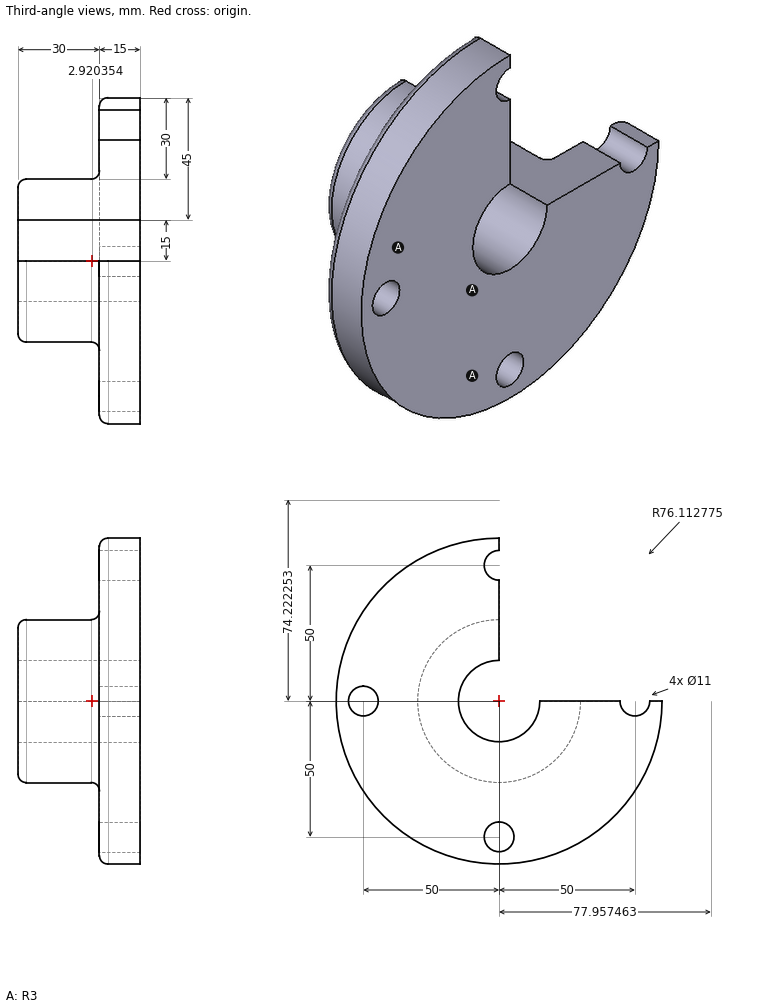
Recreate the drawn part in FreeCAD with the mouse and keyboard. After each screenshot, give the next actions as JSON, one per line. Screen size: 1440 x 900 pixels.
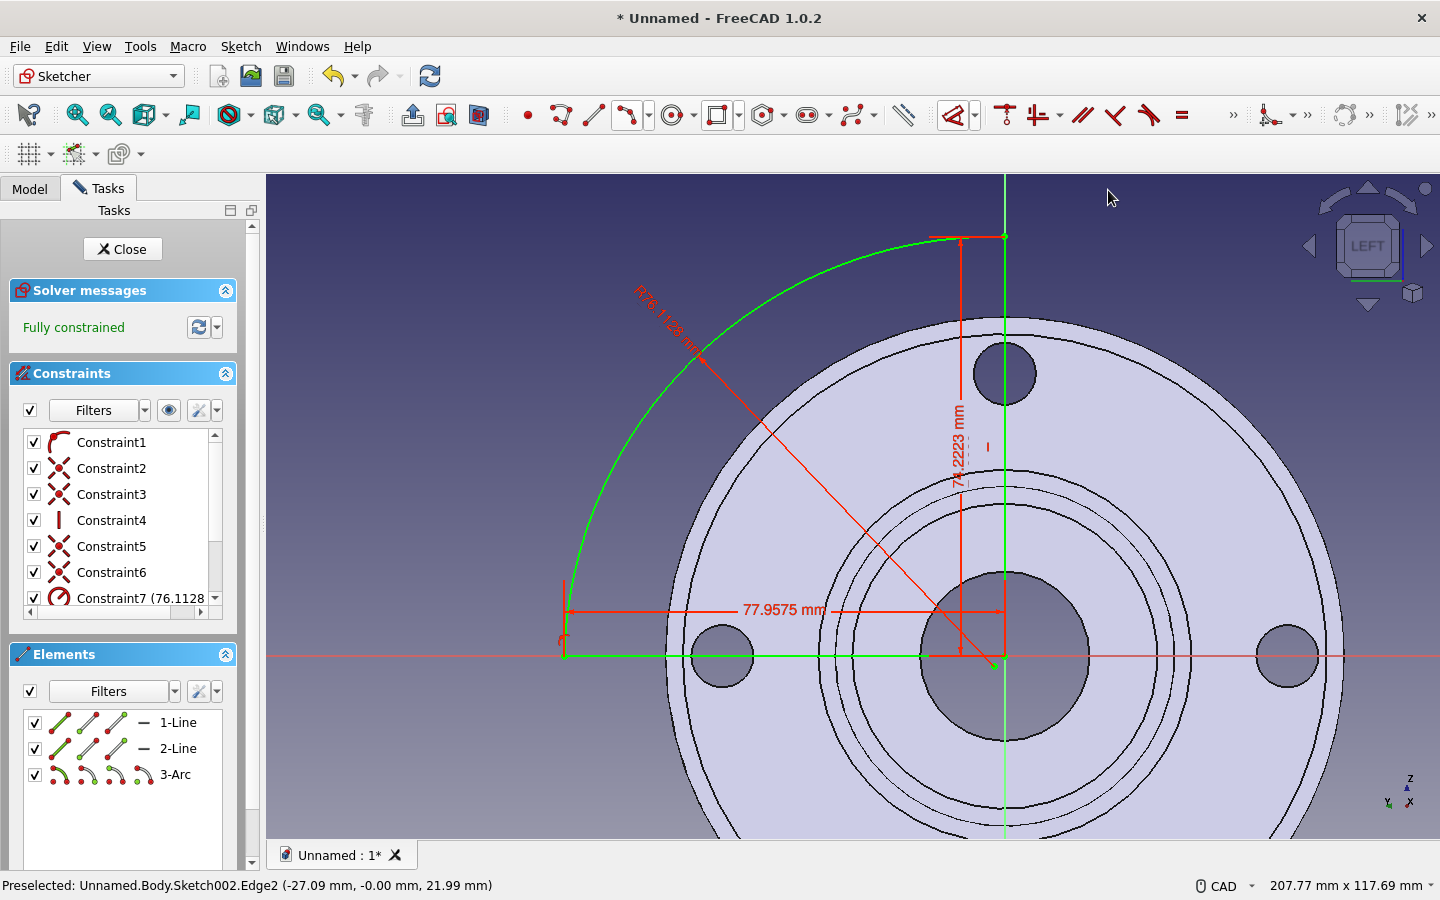
{"action": "left_click", "coordinate": [123, 249]}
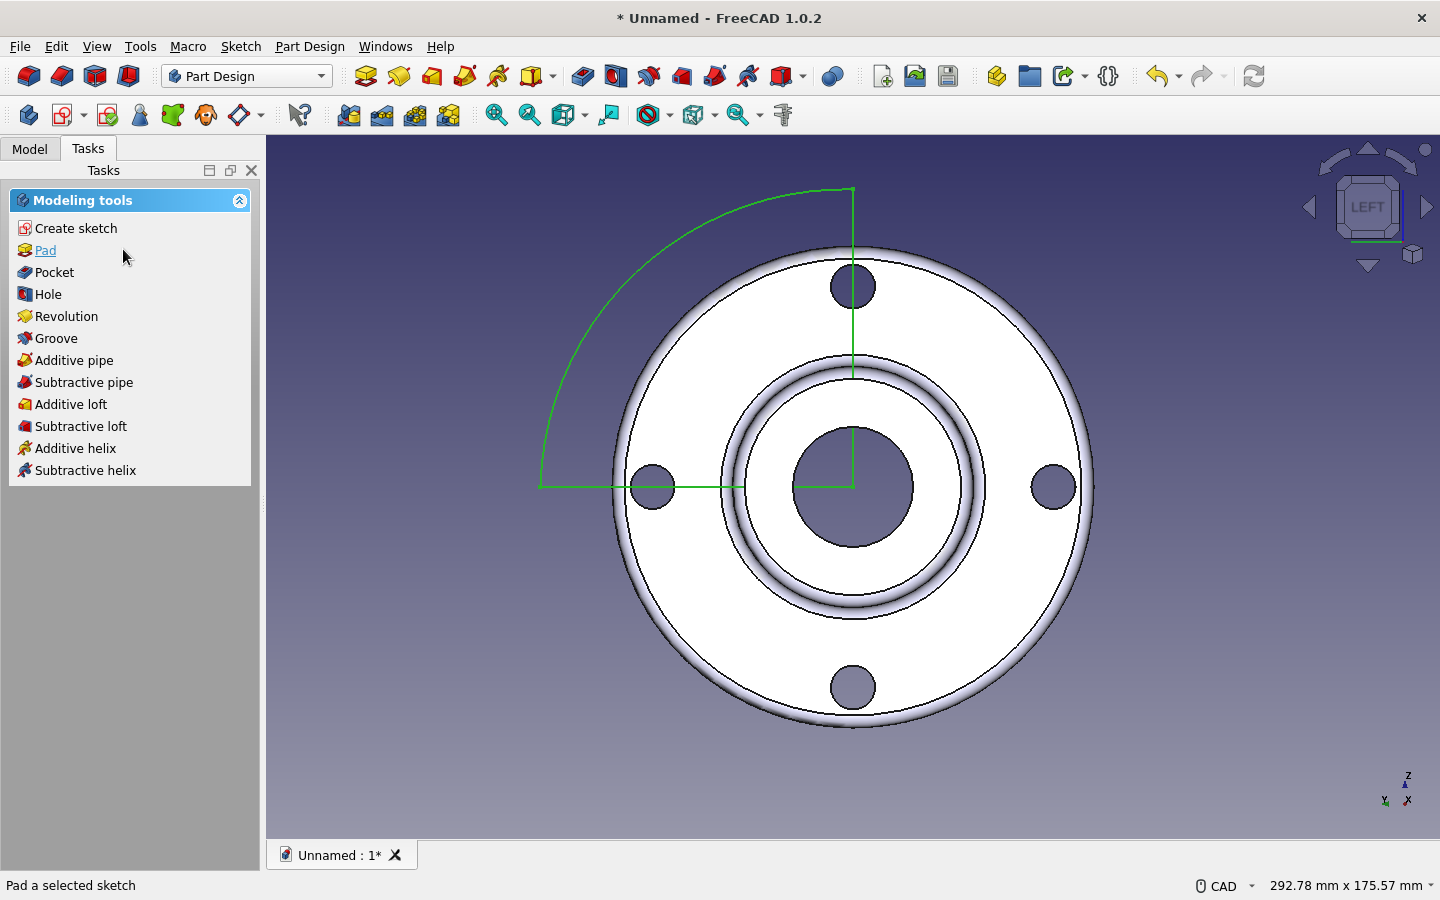
{"action": "left_click", "coordinate": [583, 76]}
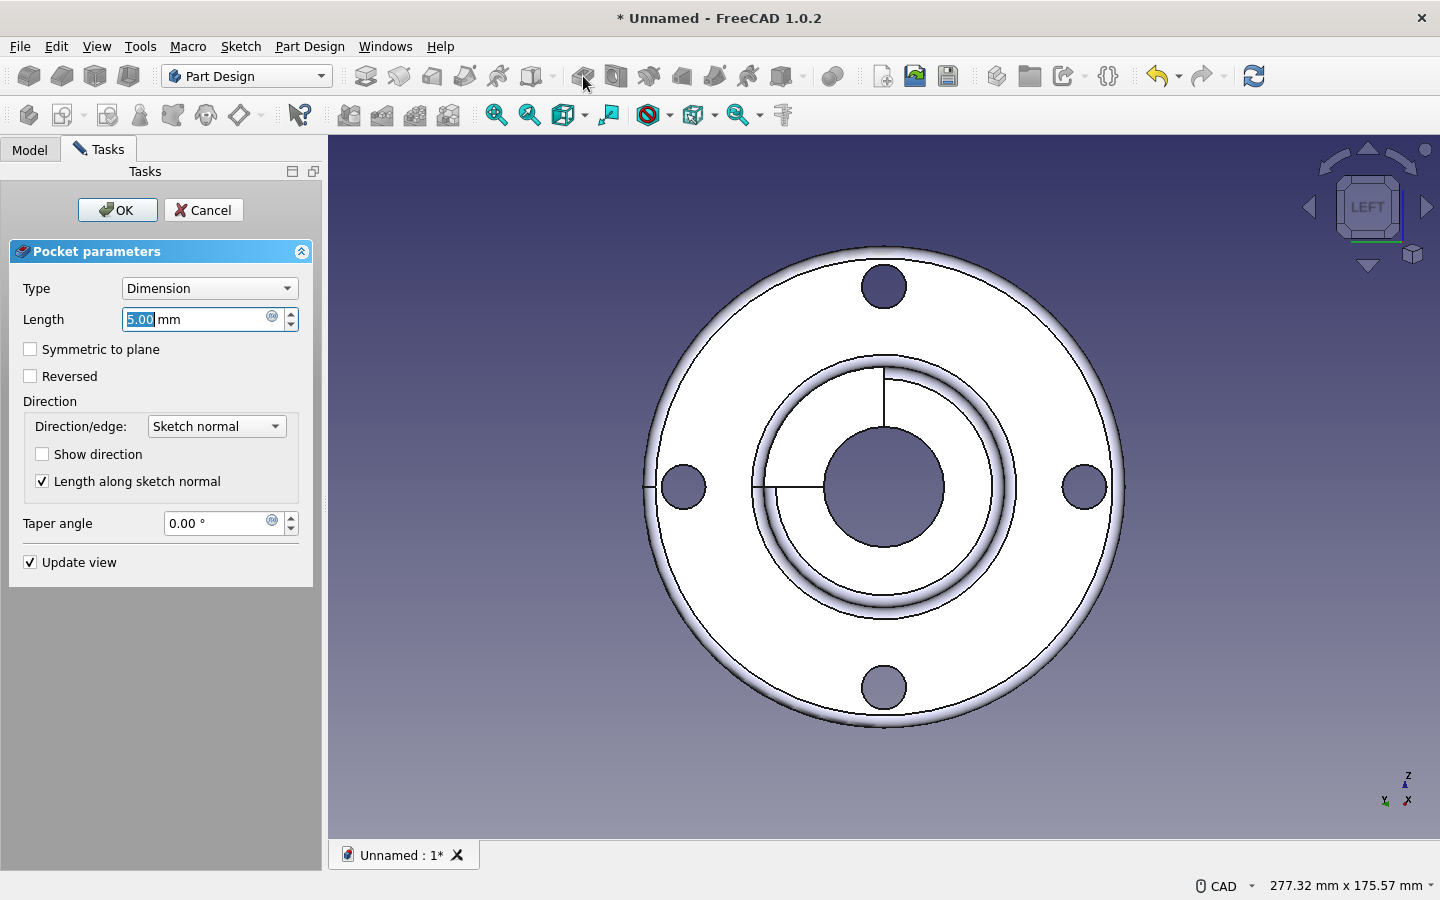
{"action": "left_click", "coordinate": [210, 288]}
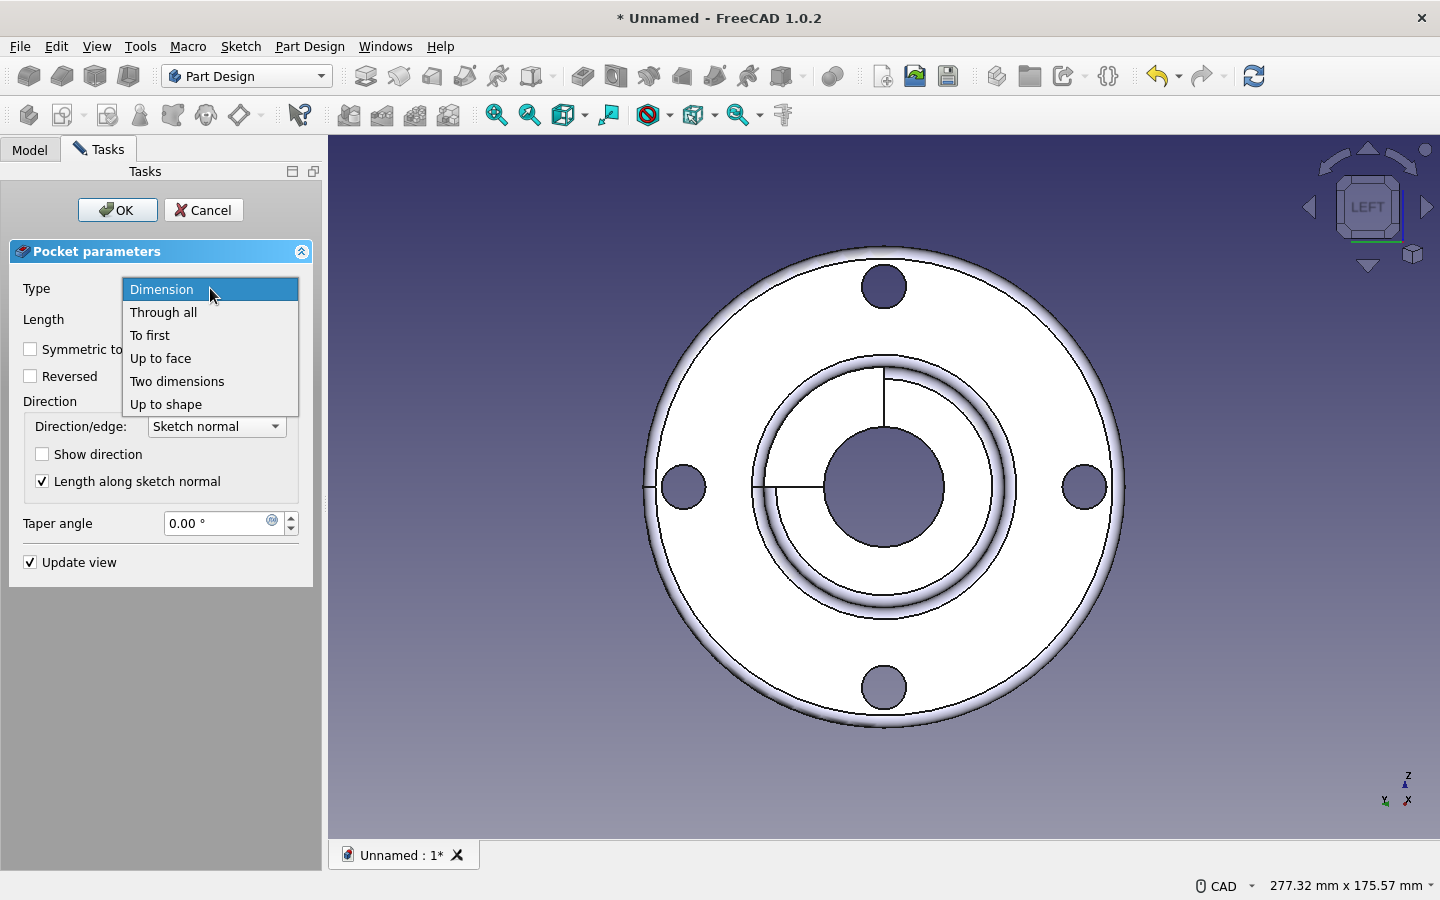
{"action": "left_click", "coordinate": [208, 312]}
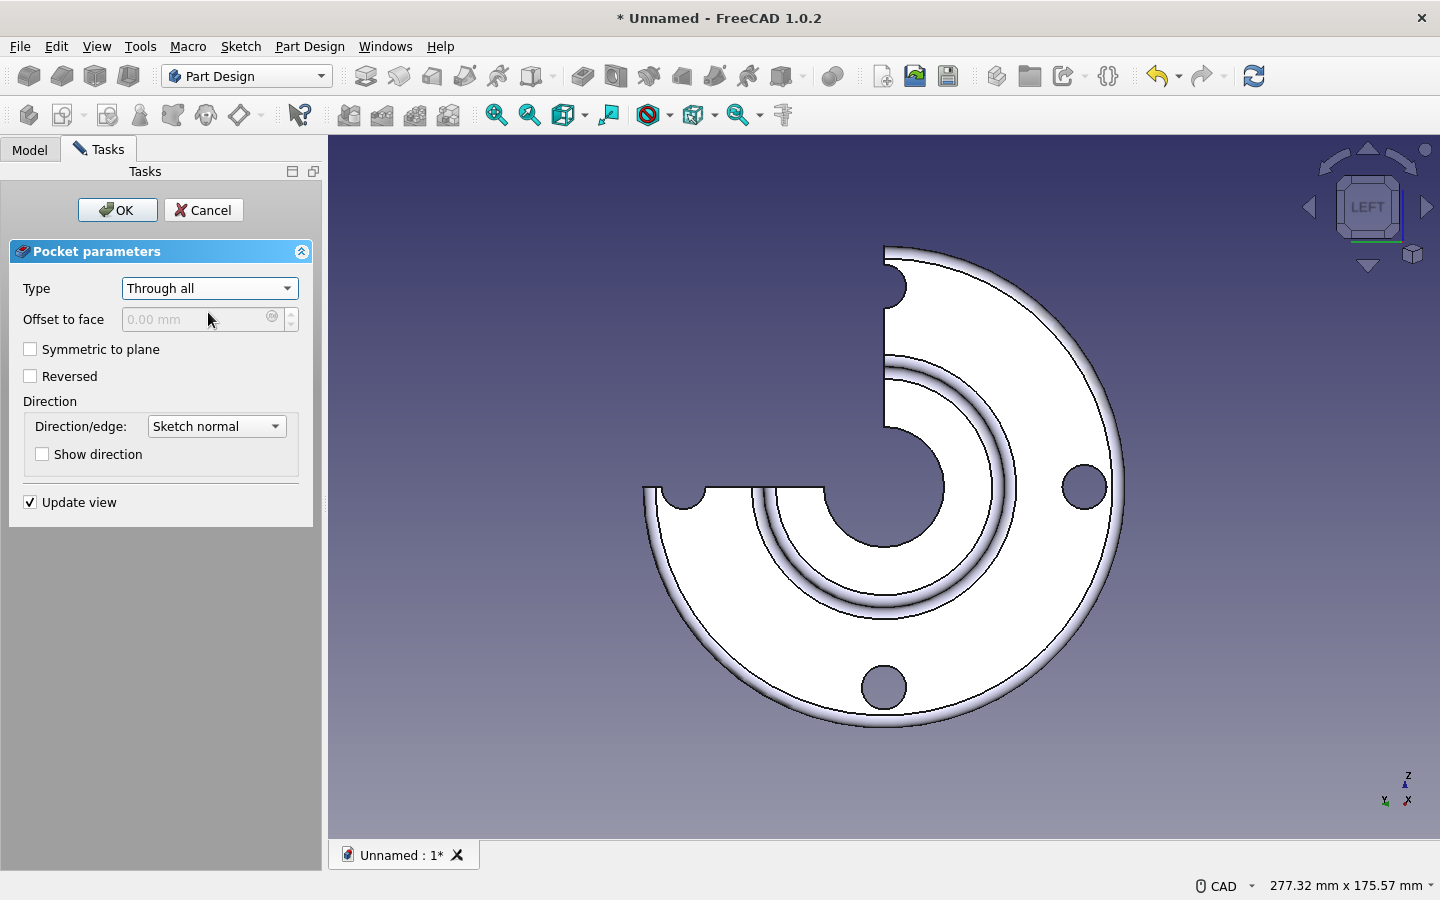
{"action": "left_click", "coordinate": [118, 210]}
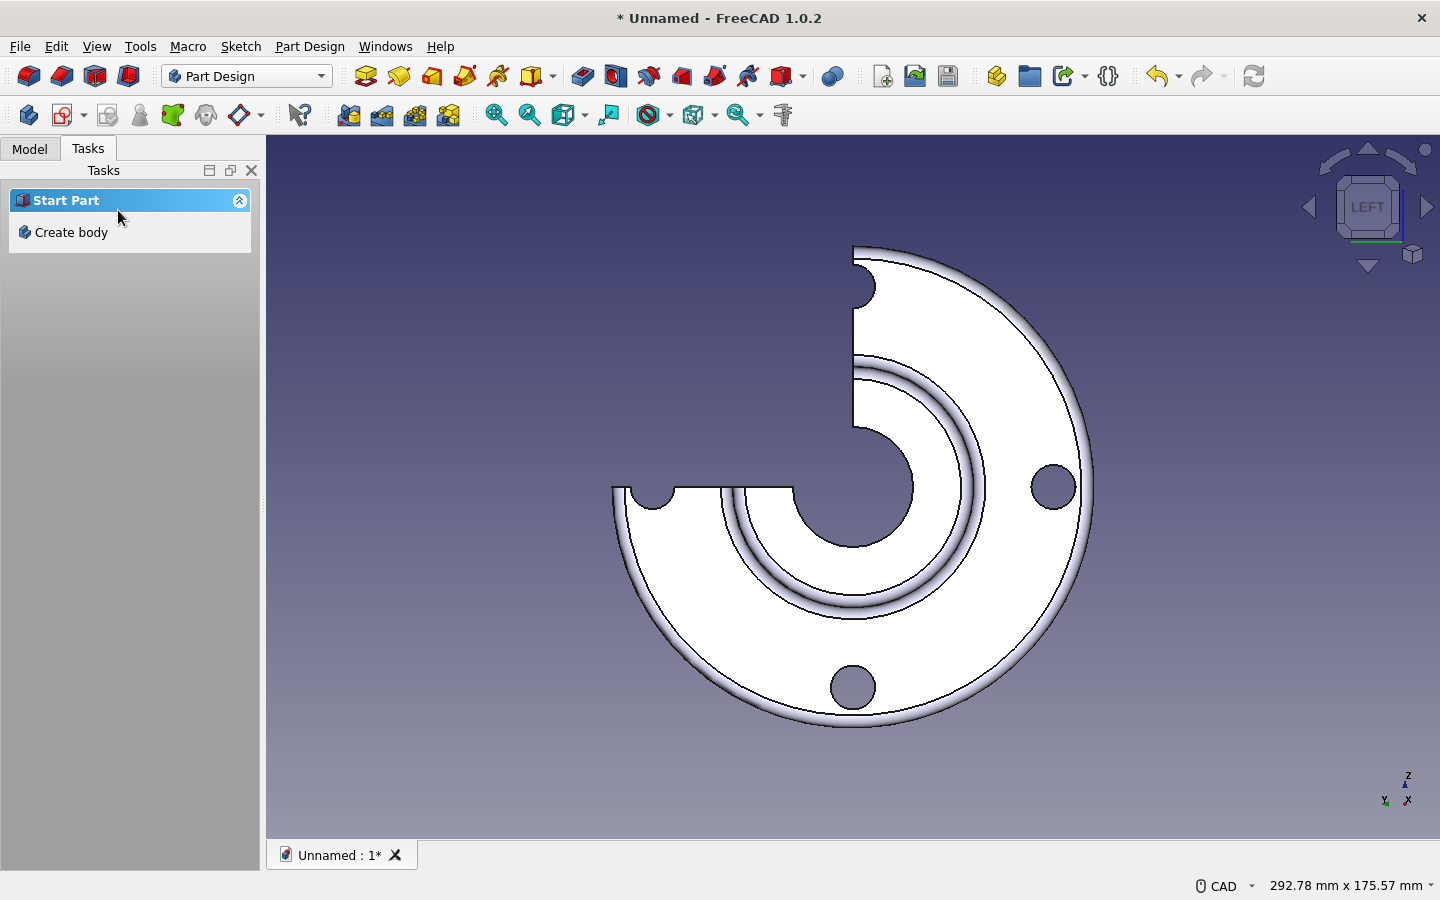
{"action": "key", "text": "0"}